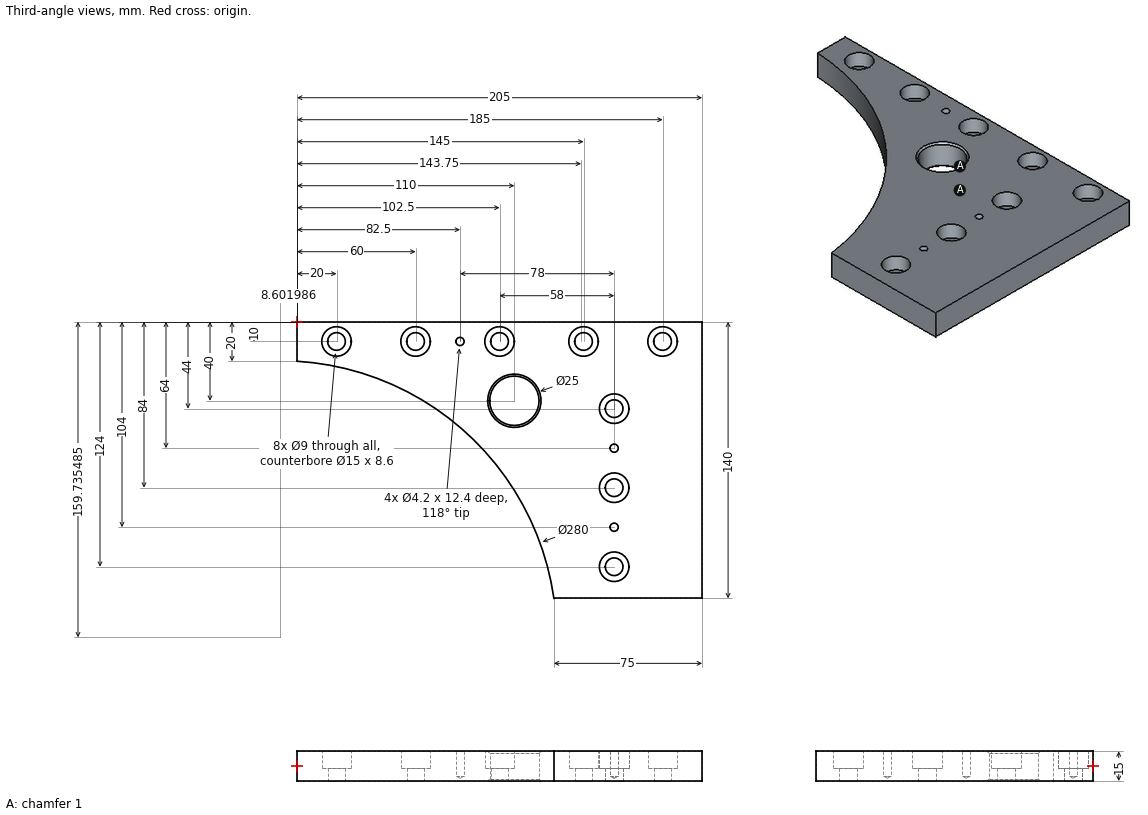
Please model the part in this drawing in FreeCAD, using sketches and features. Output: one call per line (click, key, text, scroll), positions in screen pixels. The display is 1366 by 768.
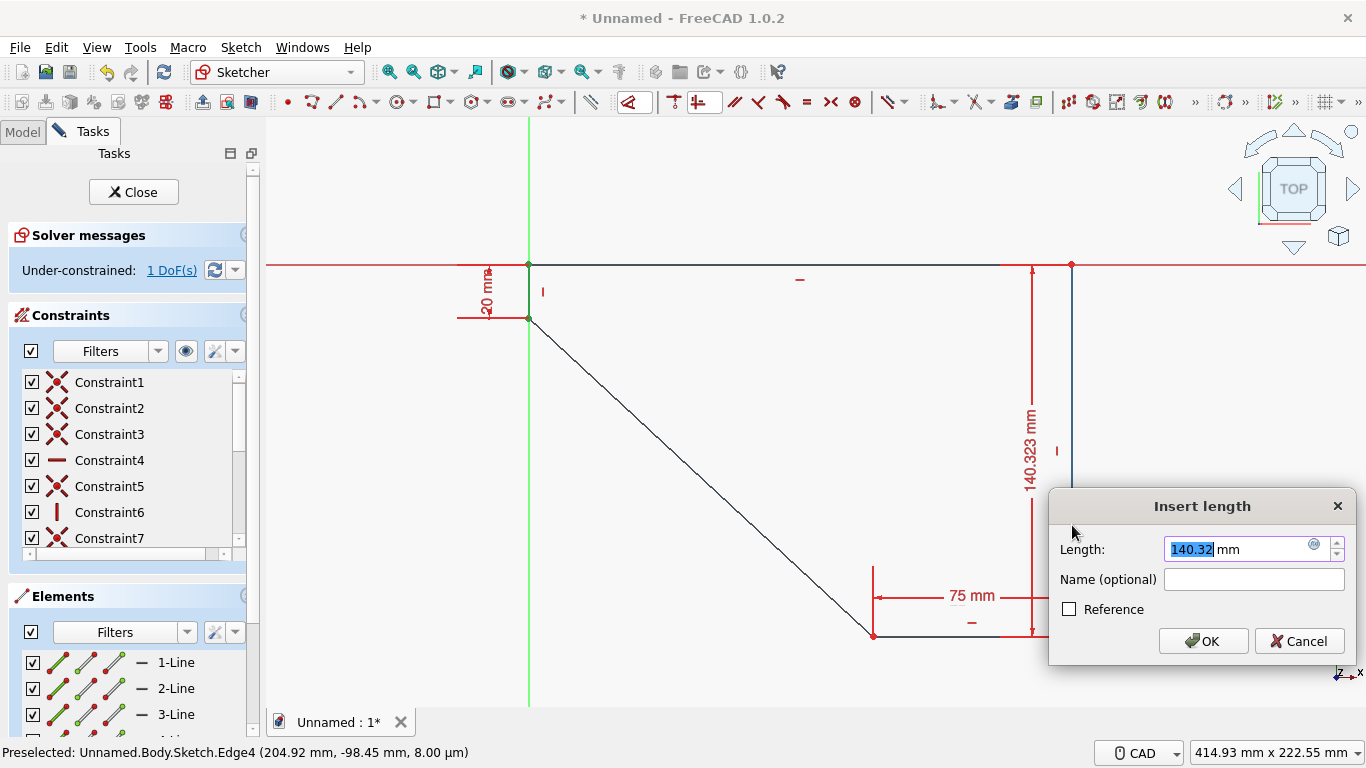
text(140)
key(Return)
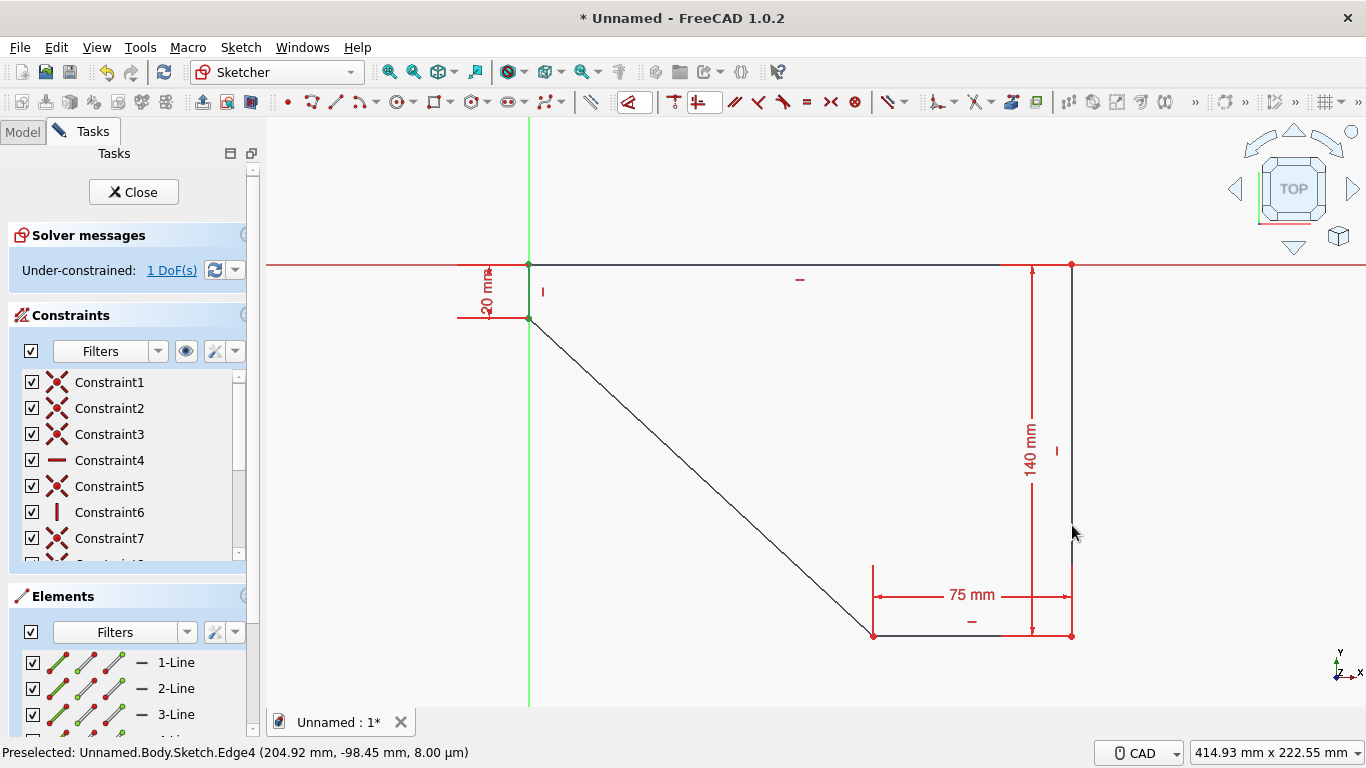
click(909, 265)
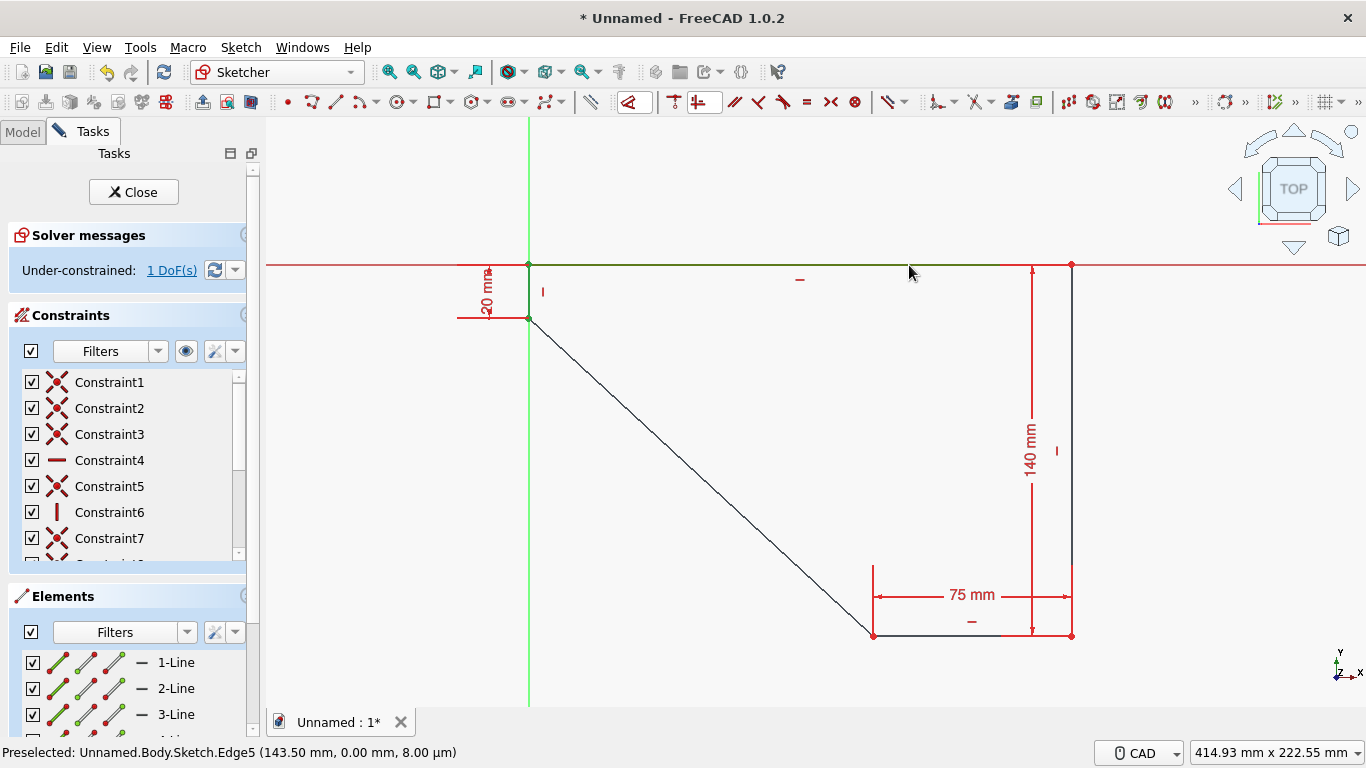
click(646, 102)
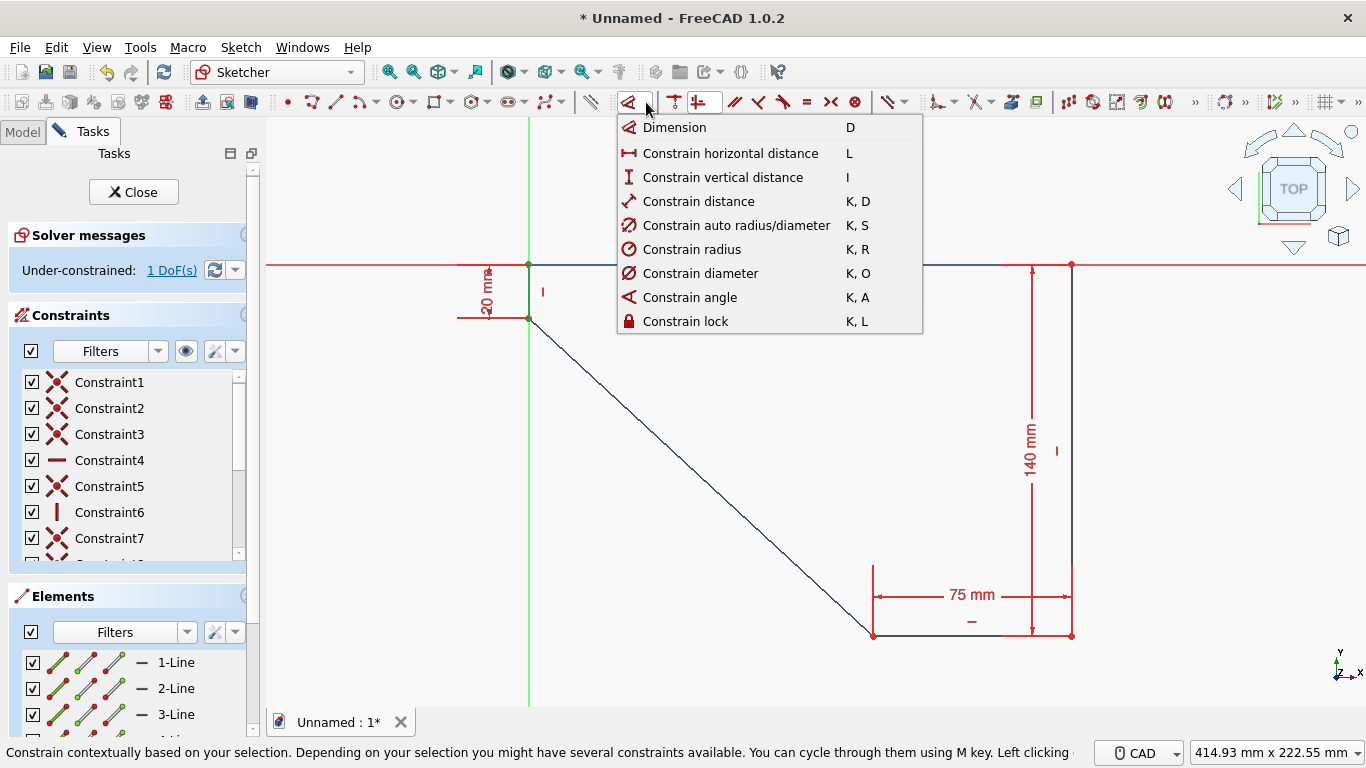
click(770, 153)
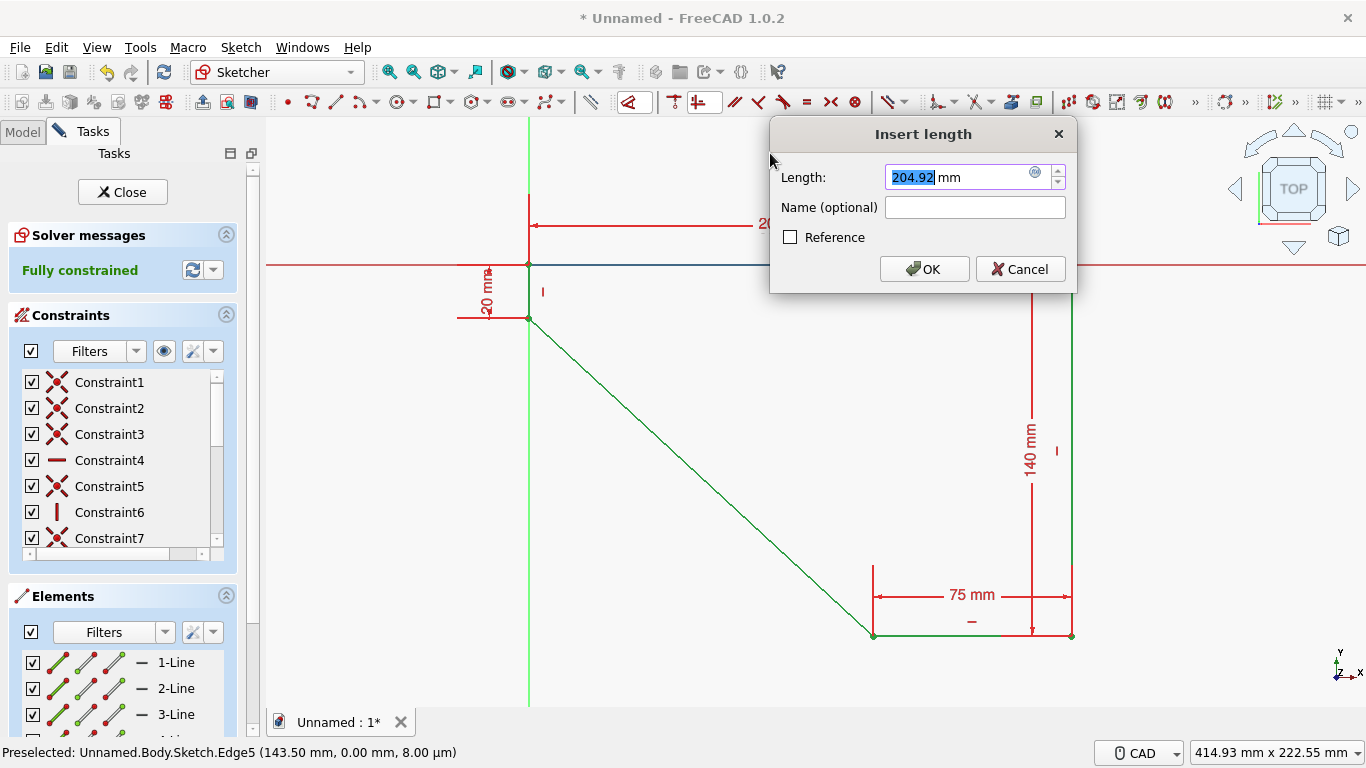
text(205)
key(Return)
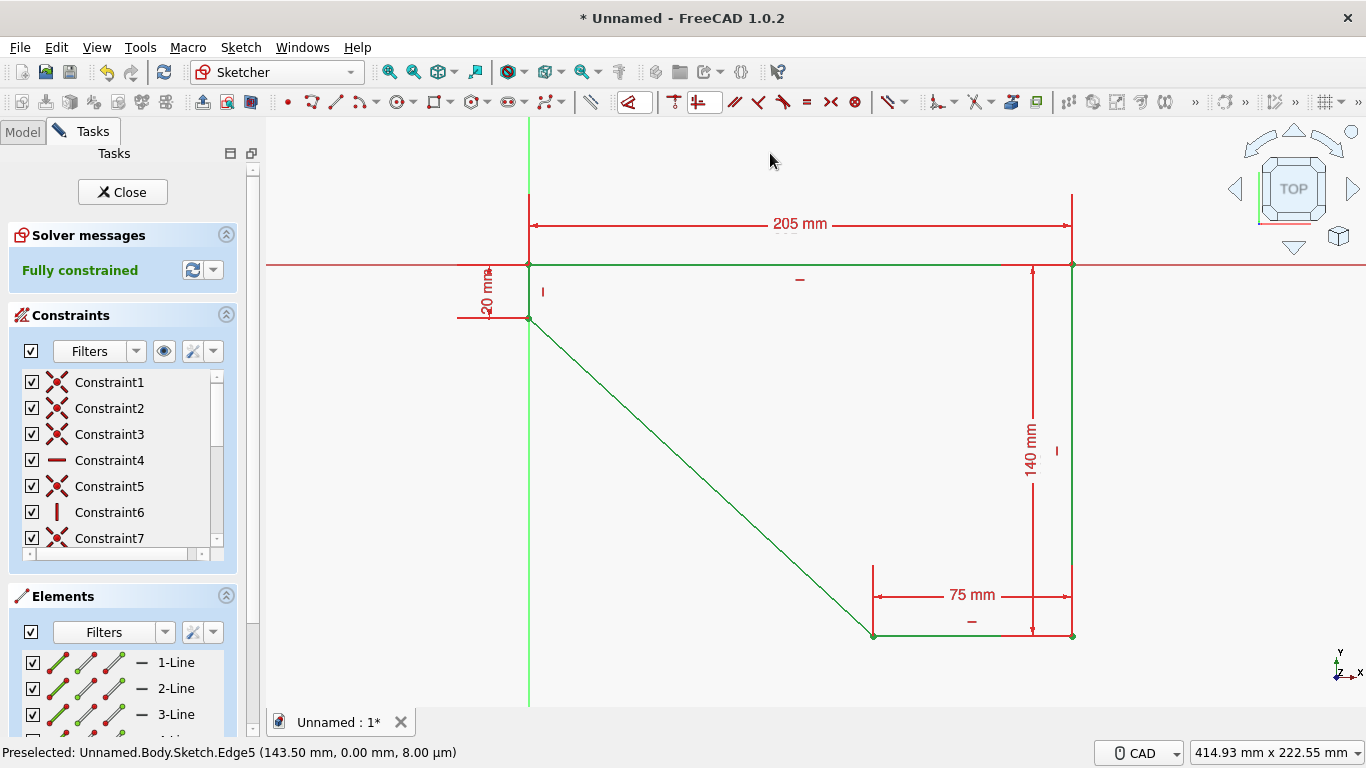
click(123, 192)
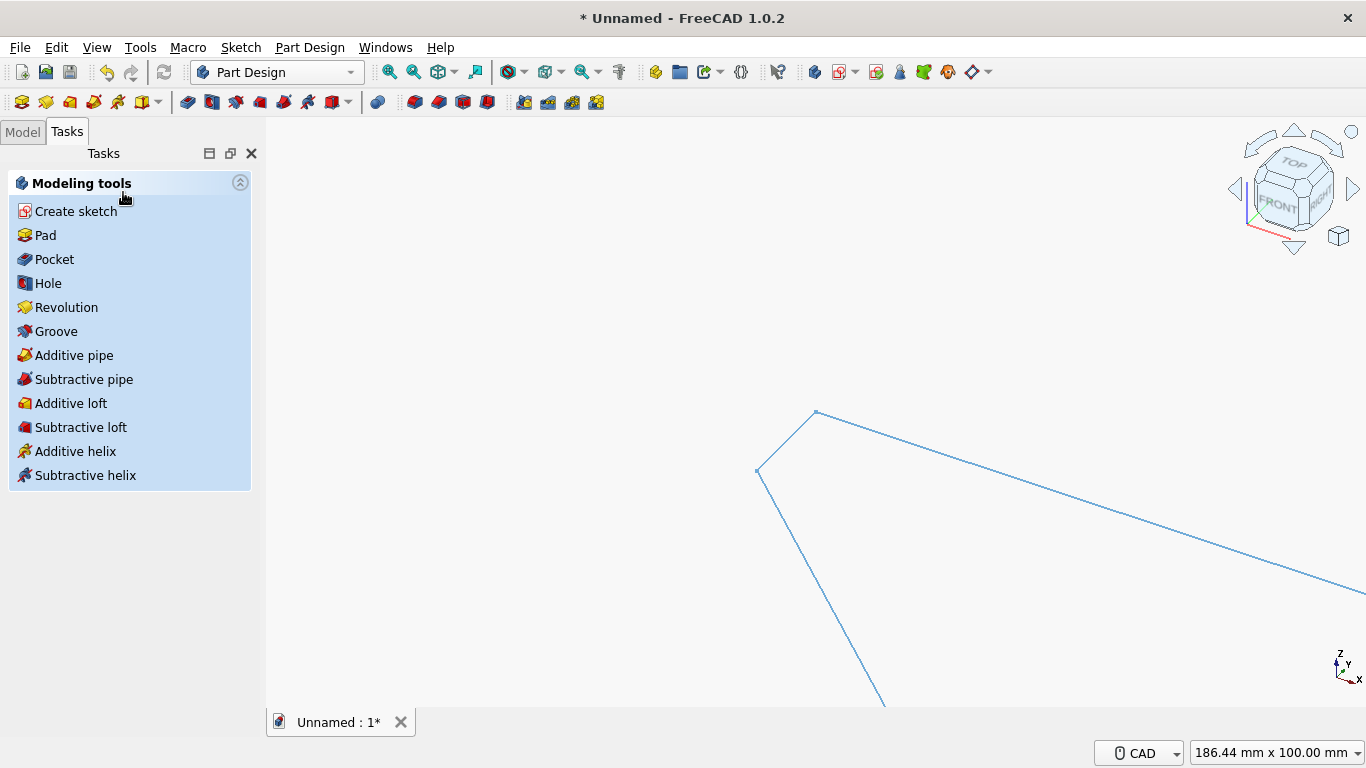
click(22, 102)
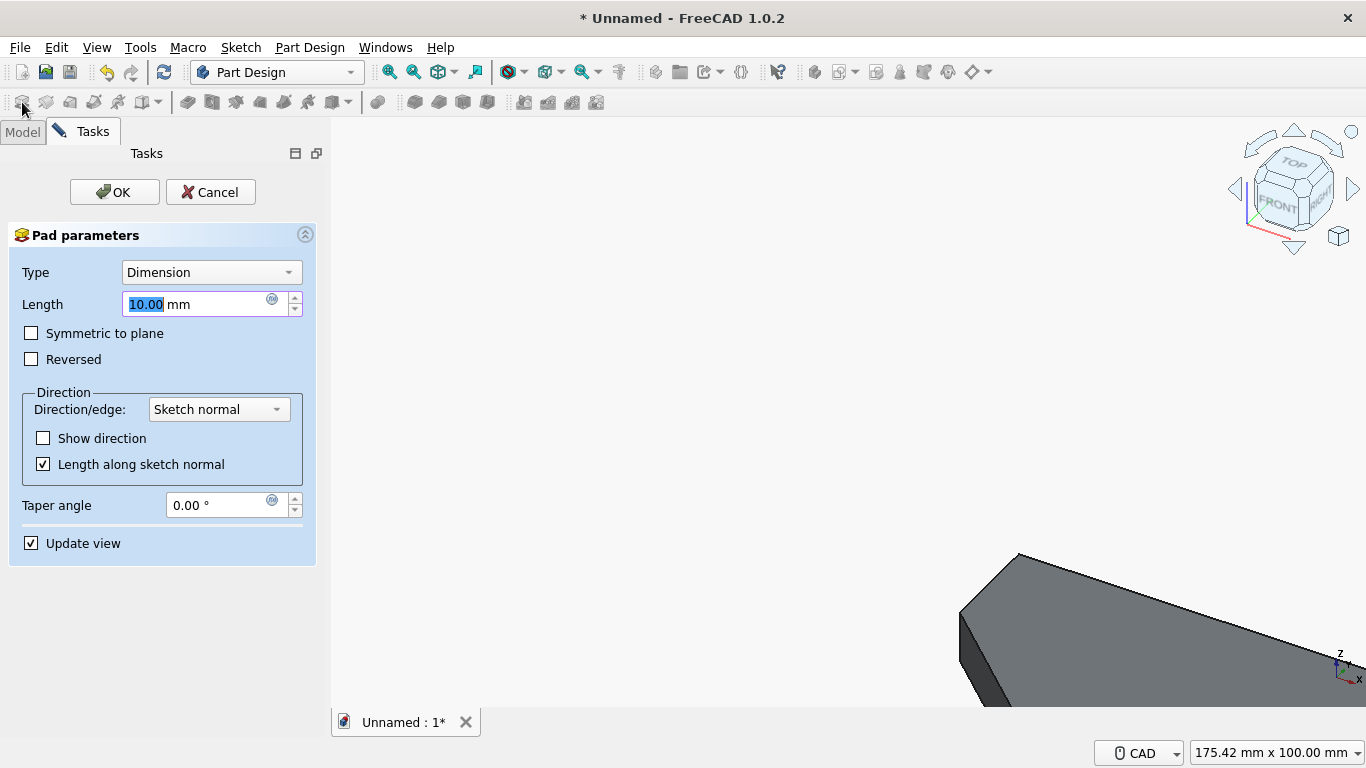
text(15)
key(Tab)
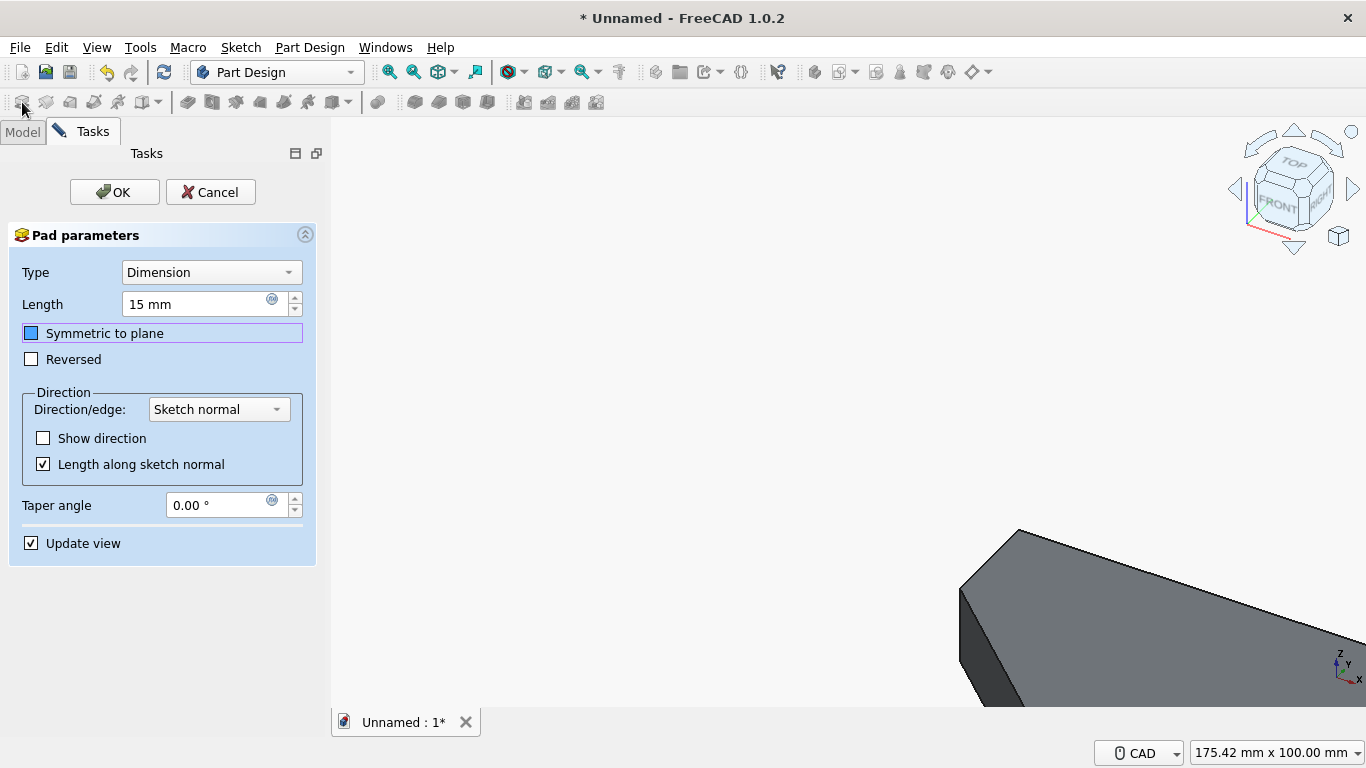
click(30, 333)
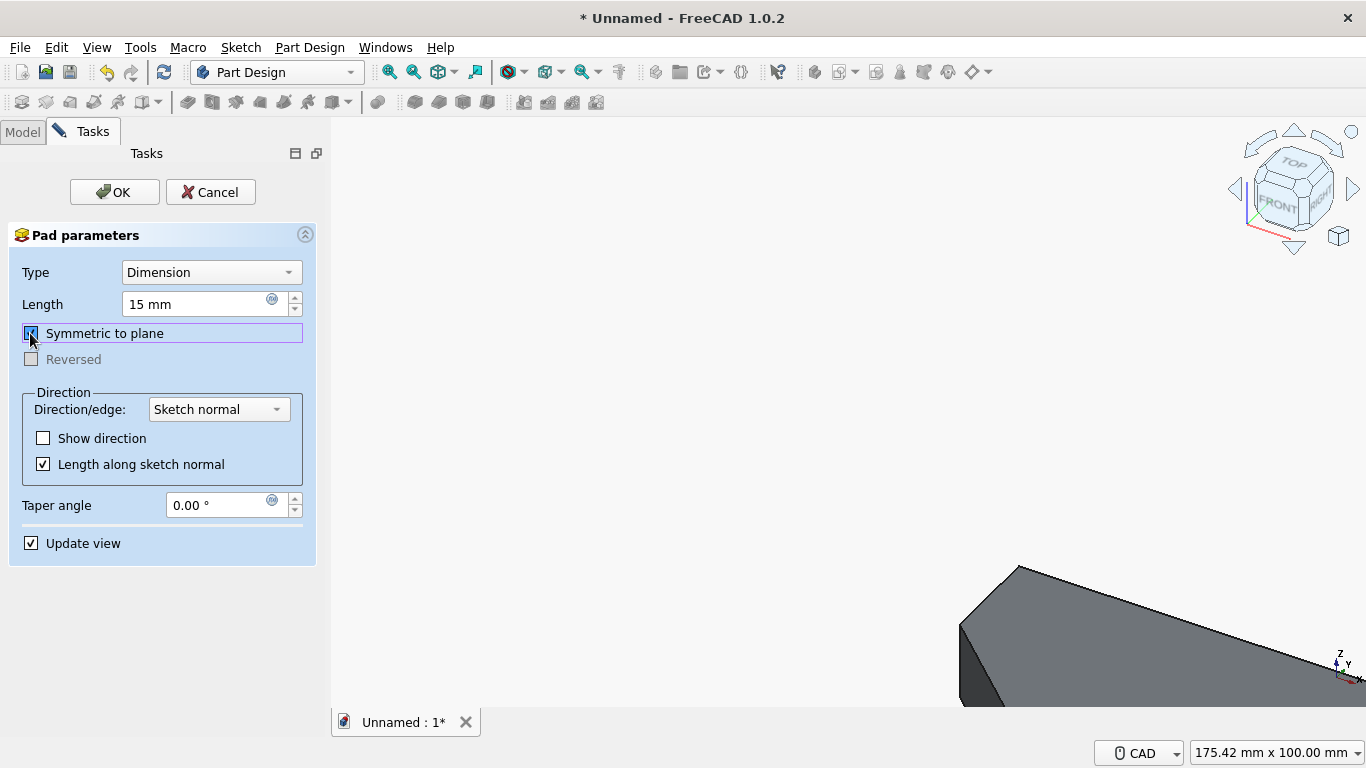
click(115, 192)